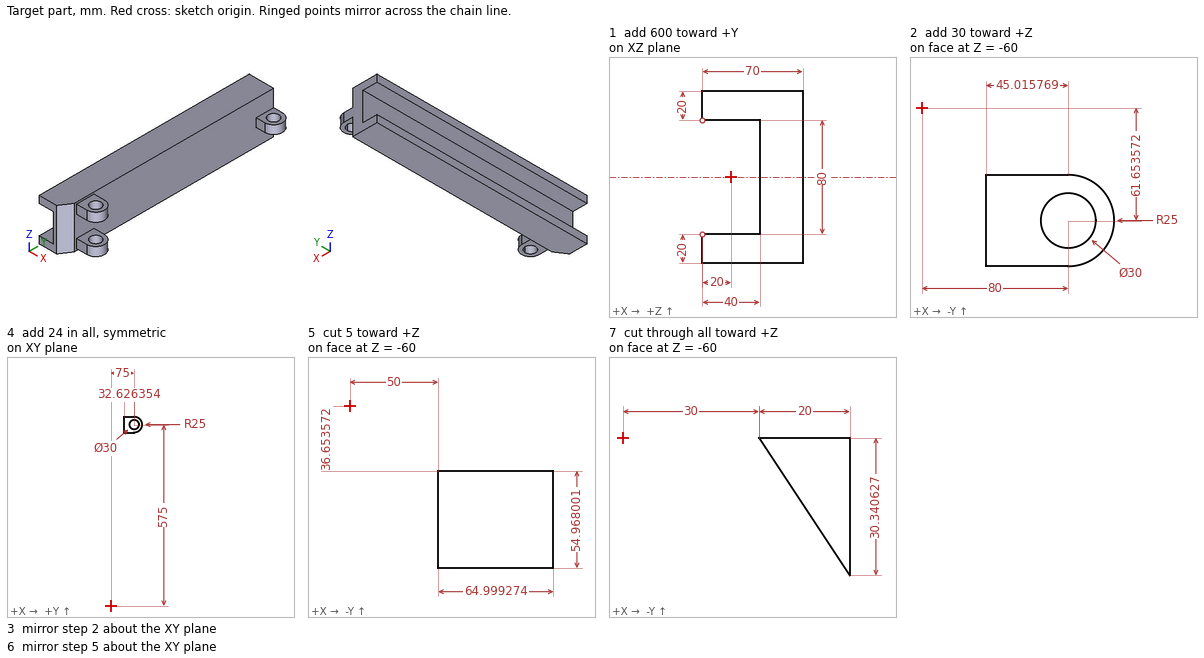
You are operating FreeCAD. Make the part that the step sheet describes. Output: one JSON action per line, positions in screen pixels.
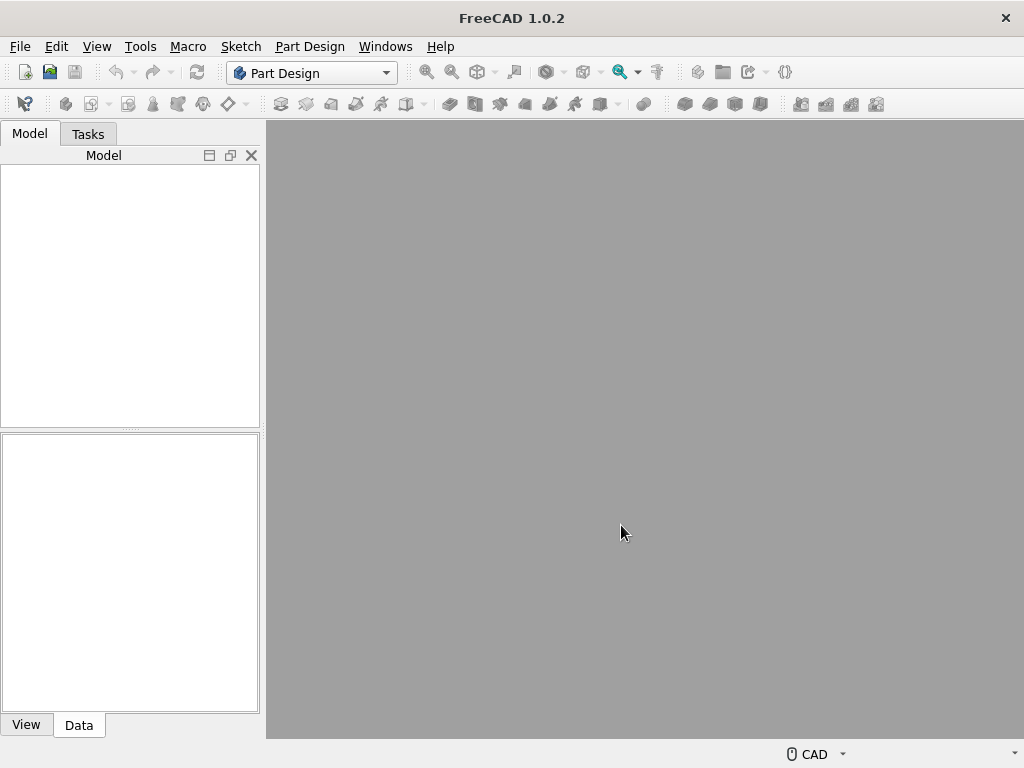
{"action": "left_click", "coordinate": [25, 72]}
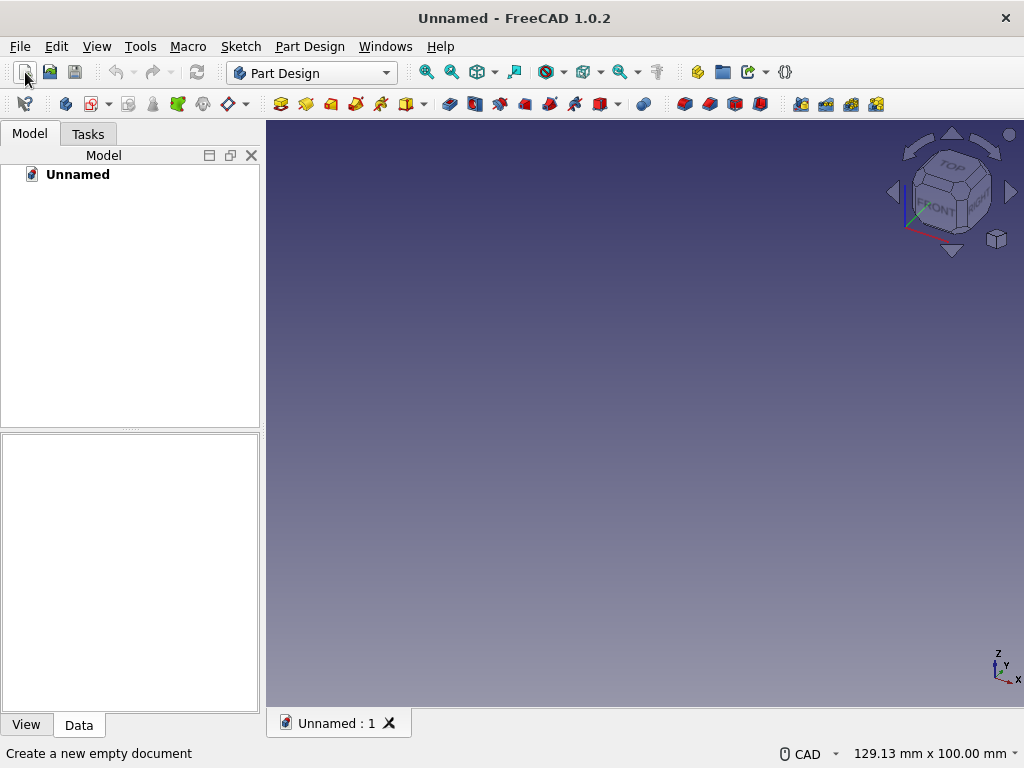
{"action": "left_click", "coordinate": [90, 104]}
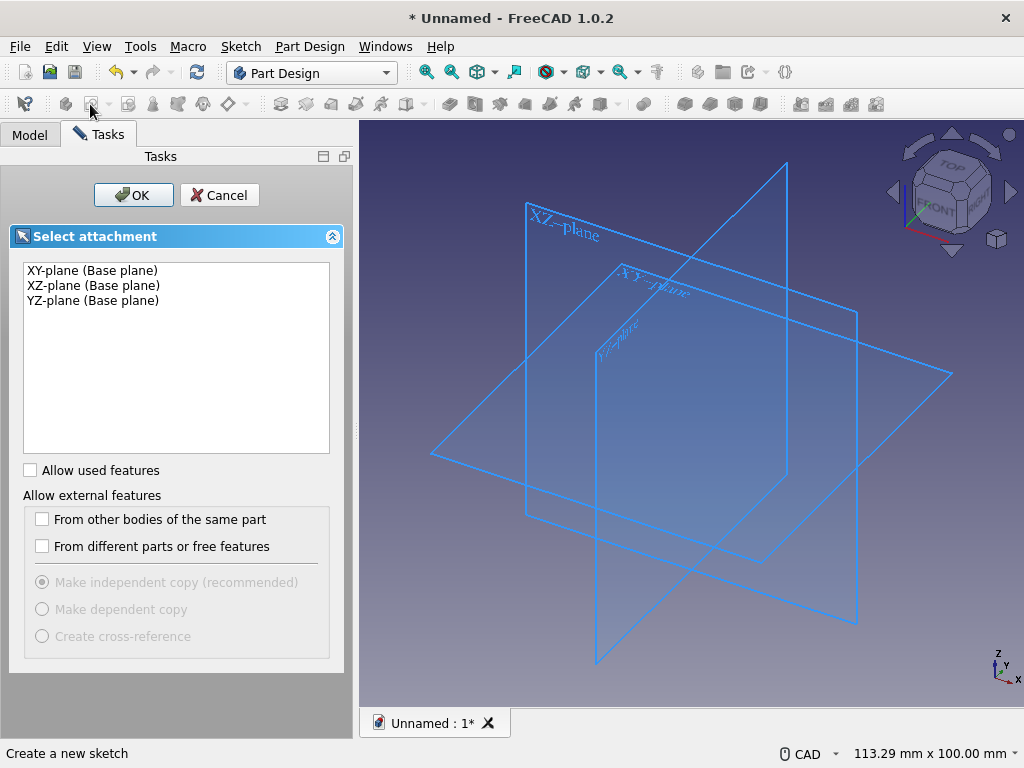
{"action": "left_click", "coordinate": [84, 286]}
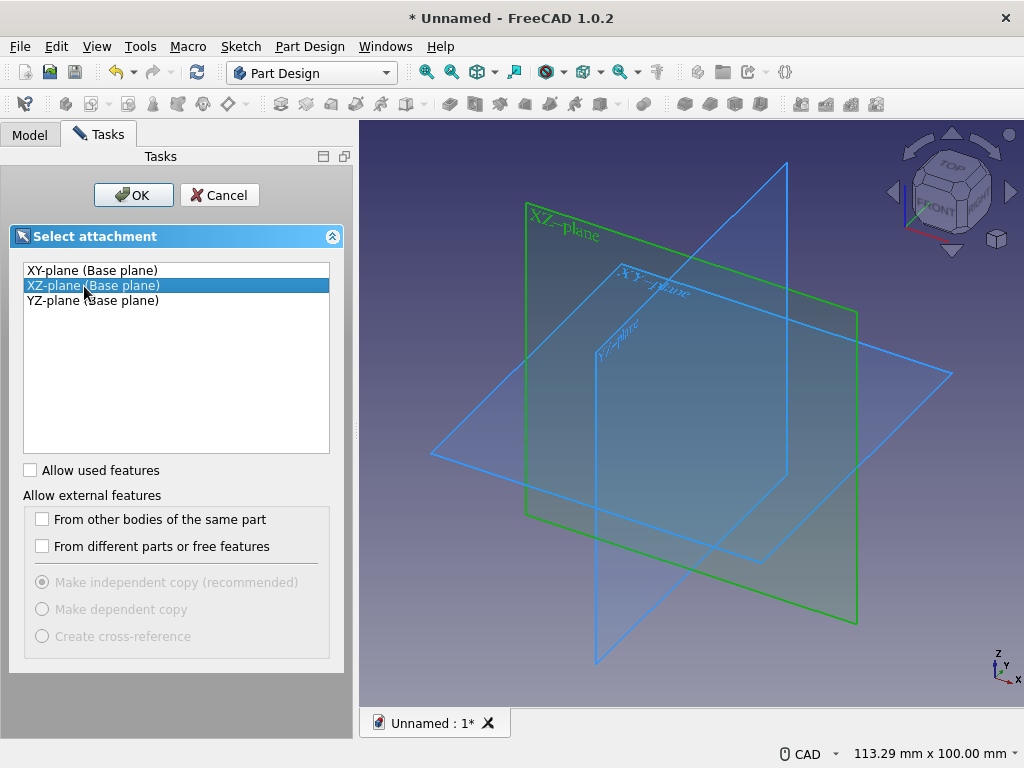
{"action": "left_click", "coordinate": [134, 195]}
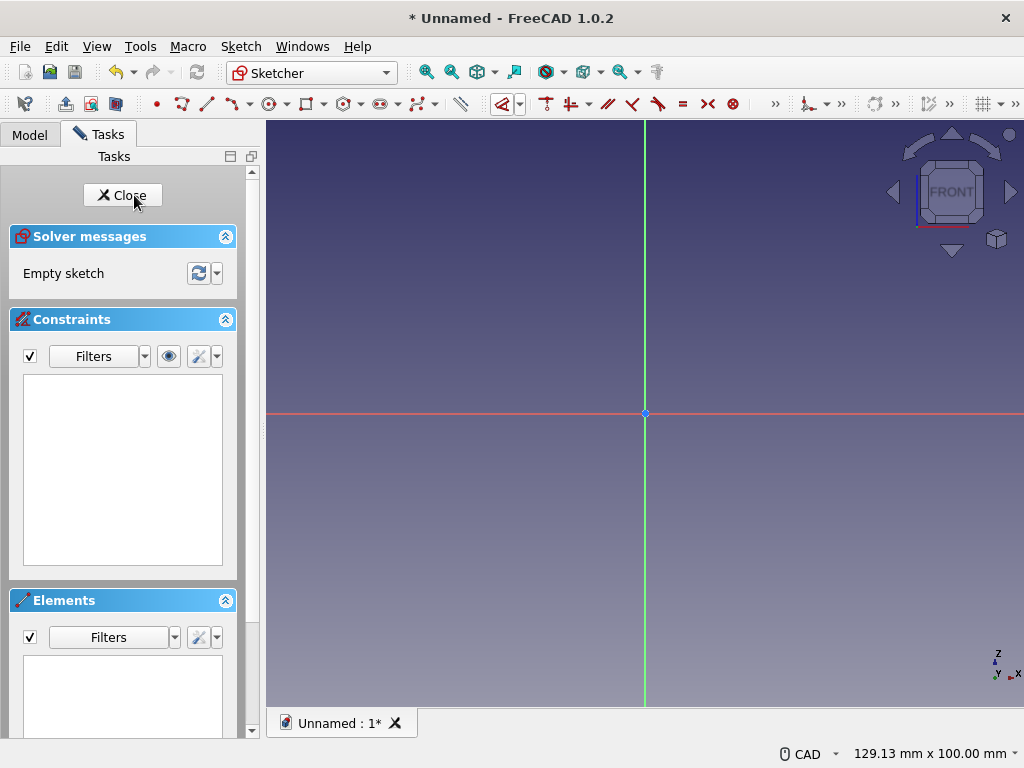
{"action": "scroll", "coordinate": [386, 414], "scroll_direction": "down", "scroll_amount": 3}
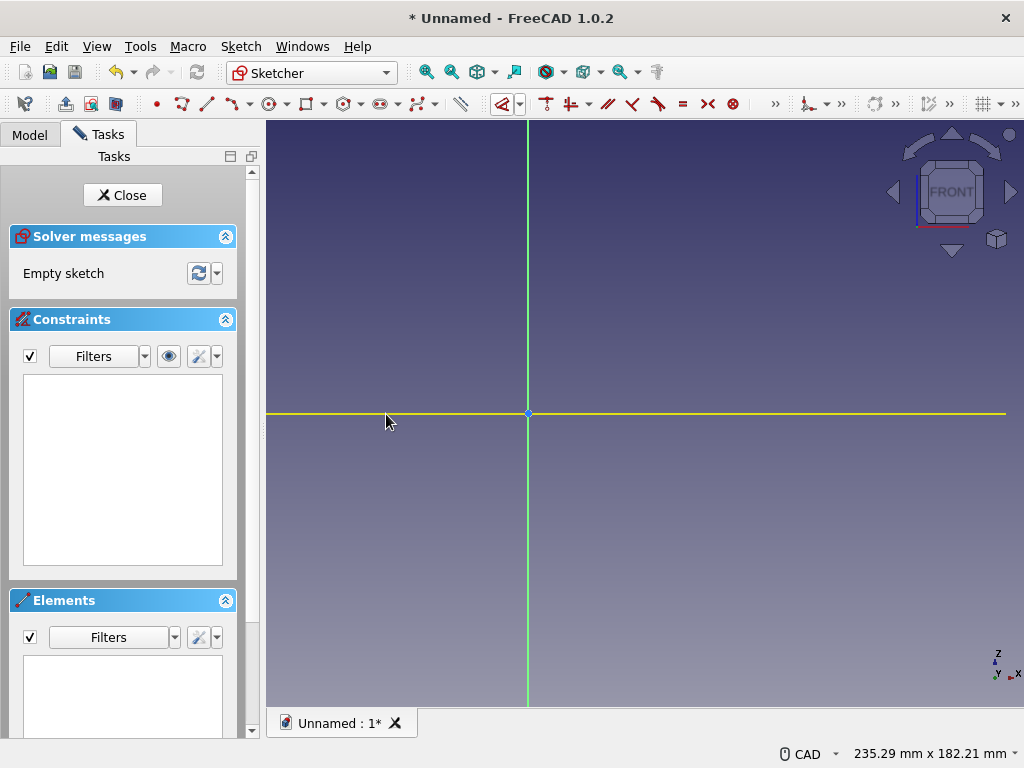
{"action": "left_click", "coordinate": [182, 104]}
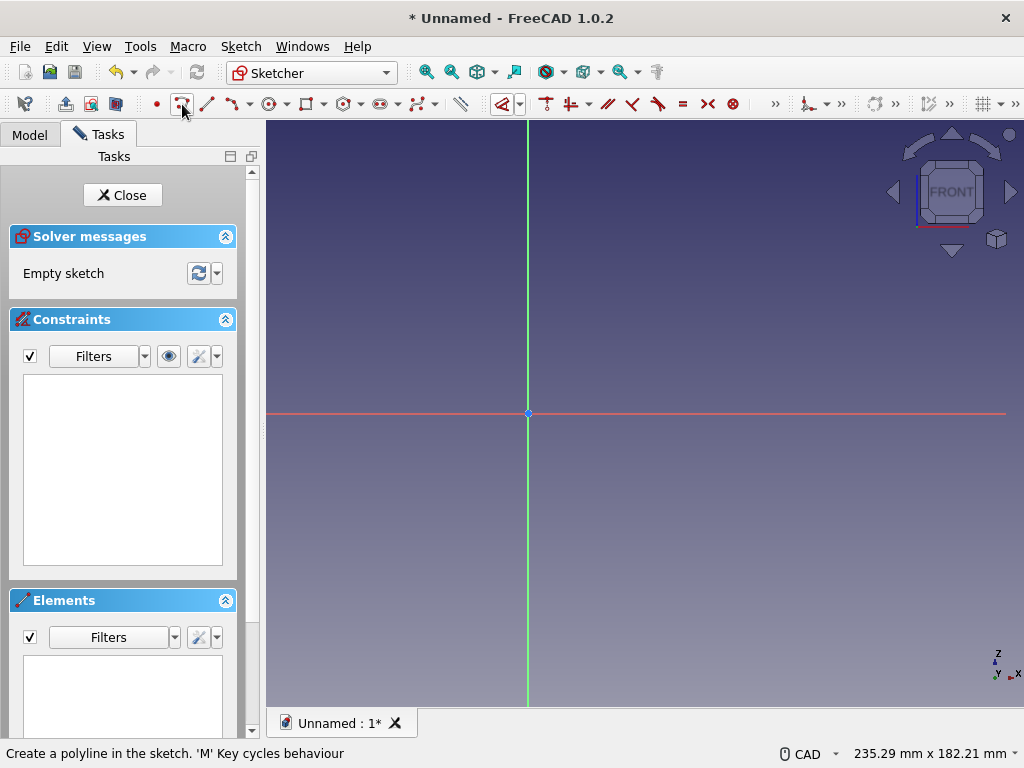
{"action": "left_click", "coordinate": [464, 543]}
{"action": "left_click", "coordinate": [593, 543]}
{"action": "left_click", "coordinate": [593, 285]}
{"action": "left_click", "coordinate": [464, 285]}
{"action": "left_click", "coordinate": [464, 221]}
{"action": "left_click", "coordinate": [689, 221]}
{"action": "left_click", "coordinate": [689, 607]}
{"action": "left_click", "coordinate": [464, 607]}
{"action": "left_click", "coordinate": [464, 544]}
{"action": "key", "text": "Escape"}
{"action": "key", "text": "Escape"}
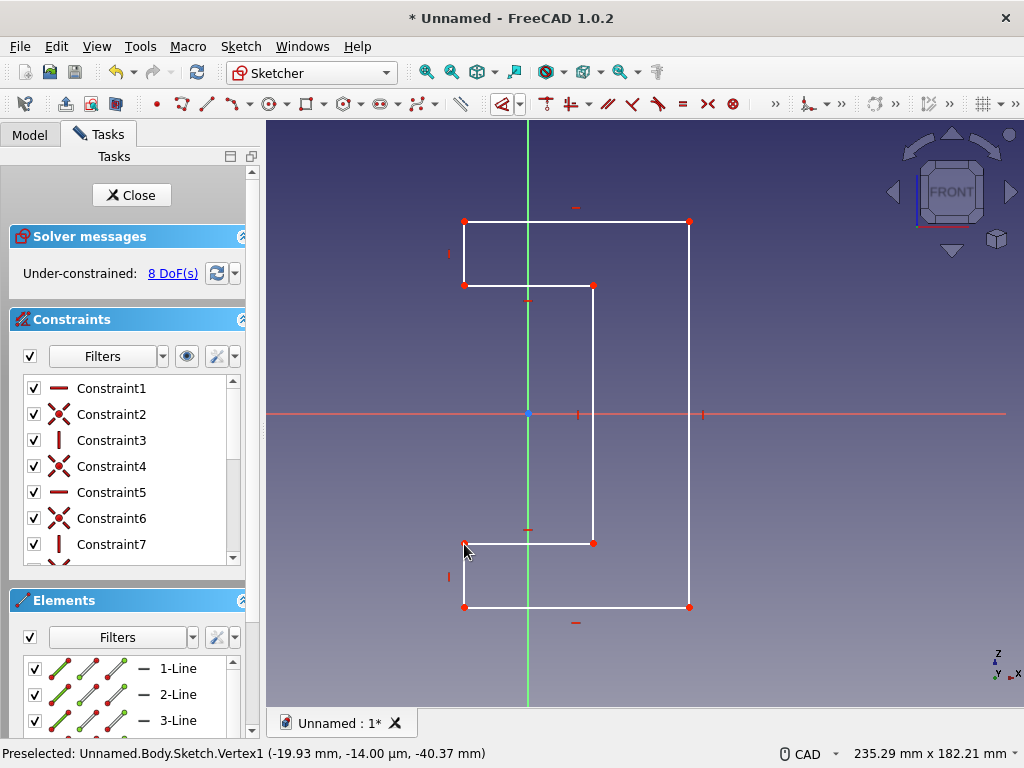
{"action": "left_click", "coordinate": [464, 544]}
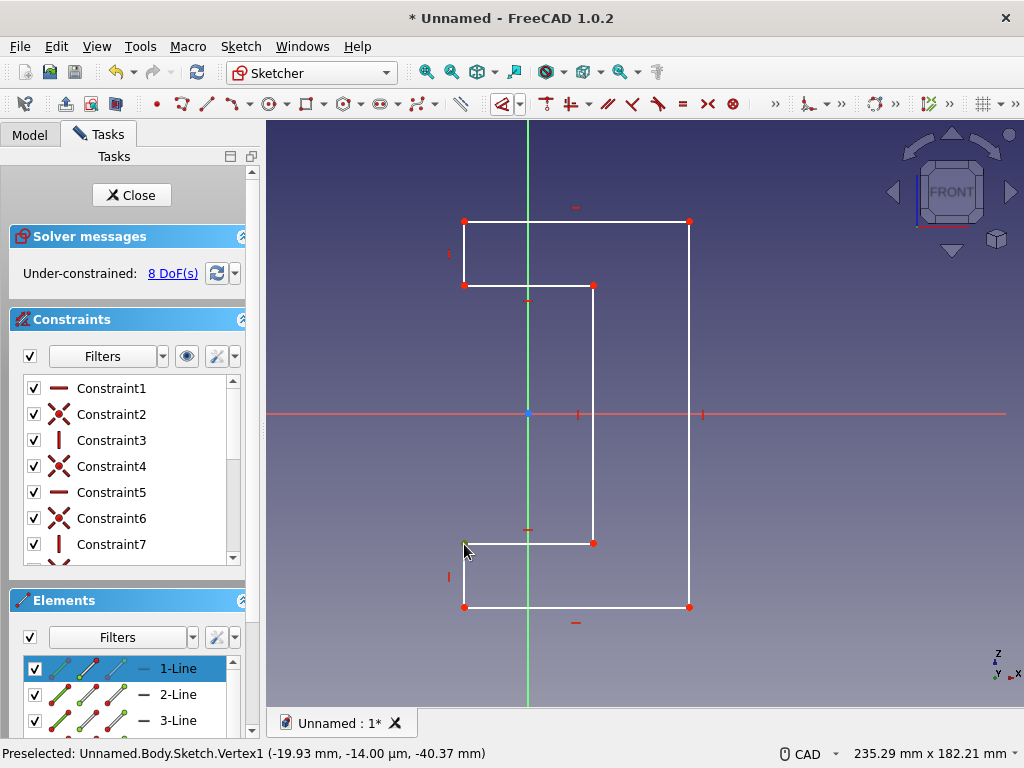
{"action": "left_click", "coordinate": [464, 286]}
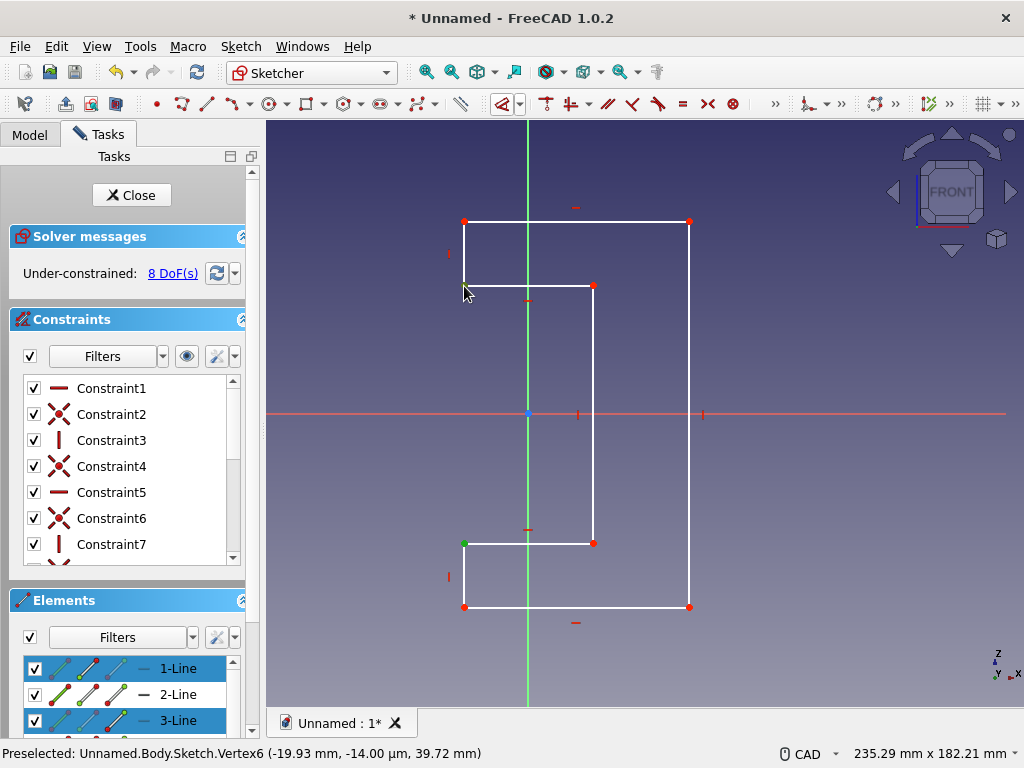
{"action": "left_click", "coordinate": [334, 414]}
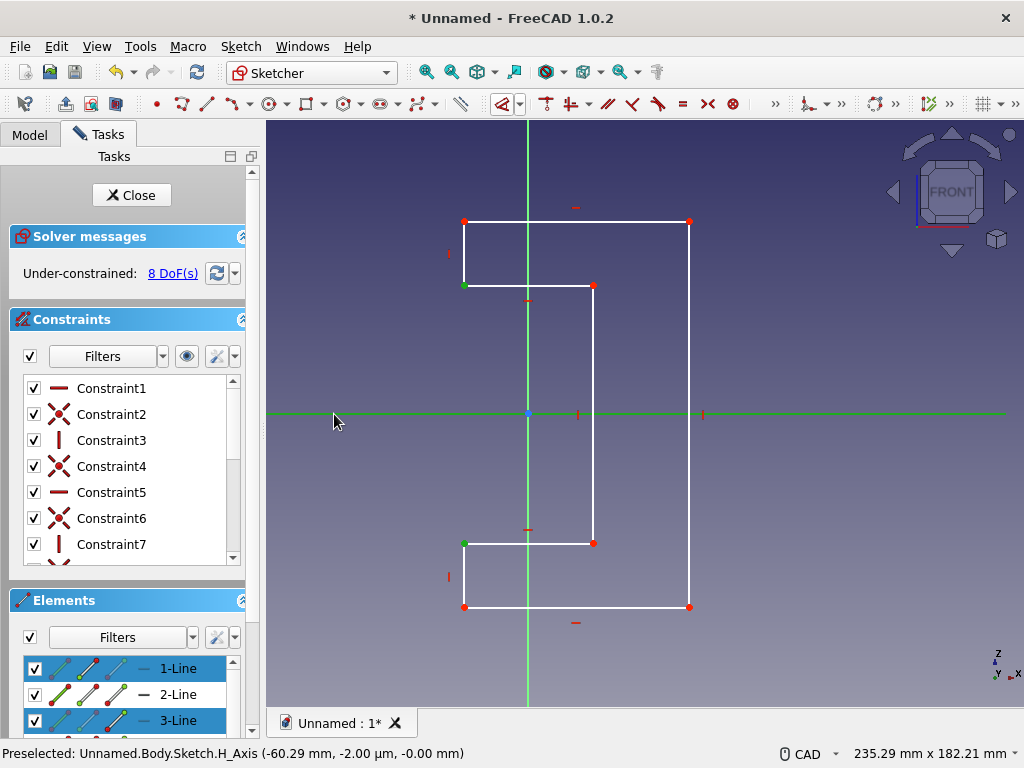
{"action": "left_click", "coordinate": [708, 104]}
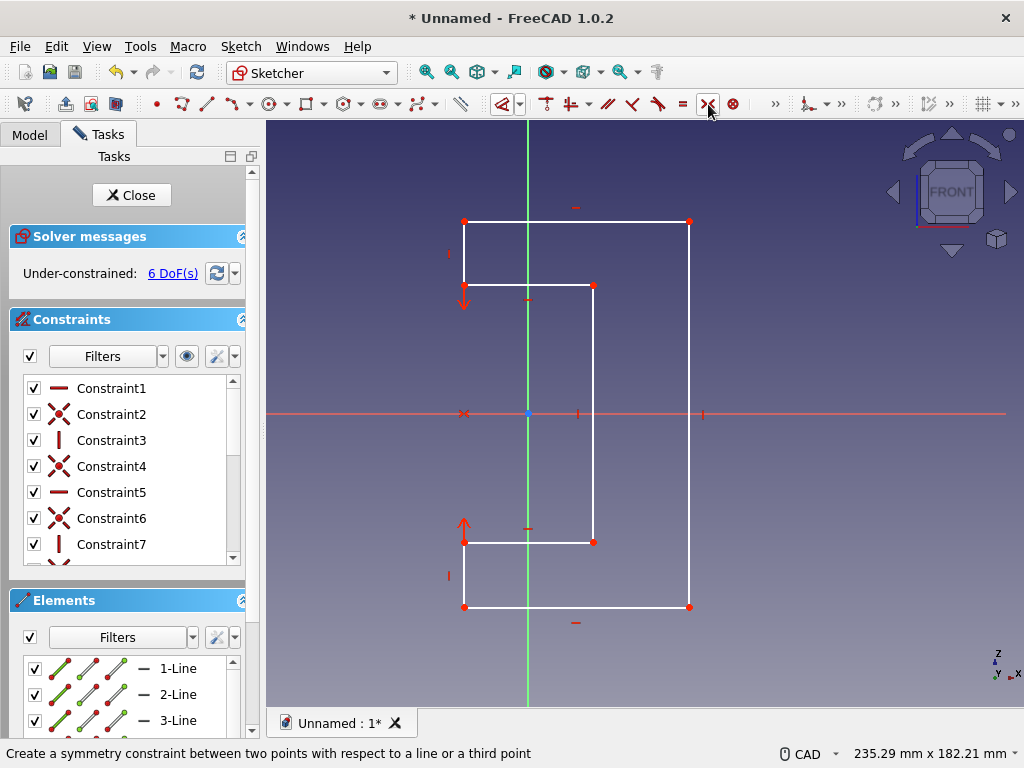
{"action": "left_click", "coordinate": [502, 104]}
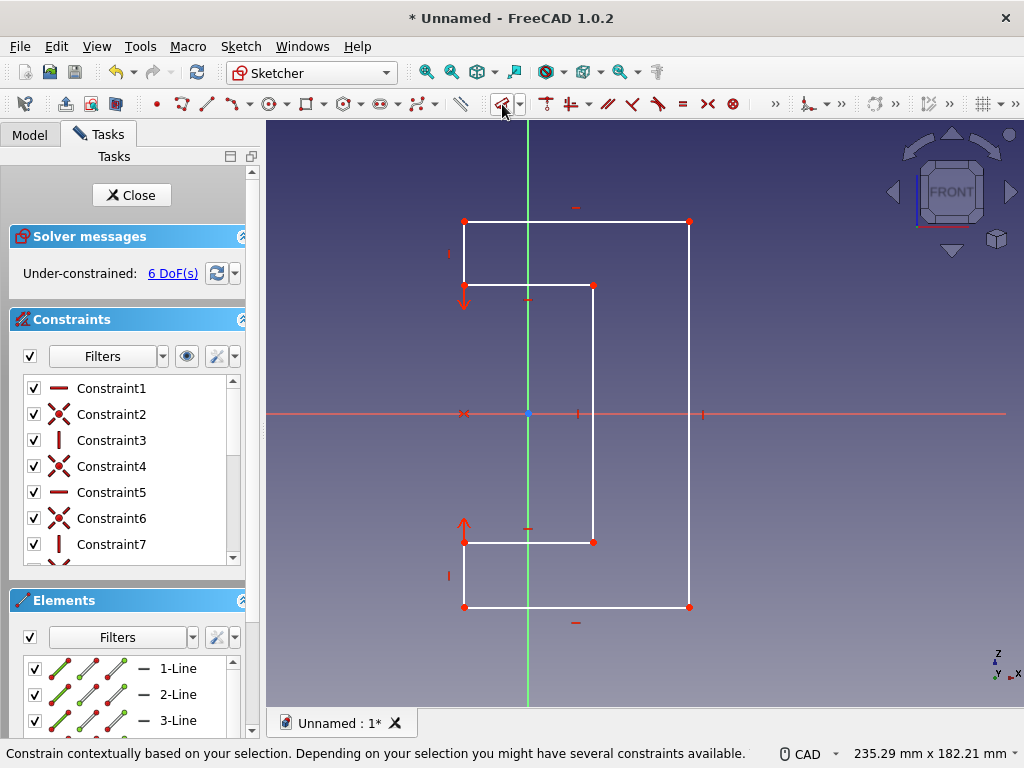
{"action": "left_click", "coordinate": [503, 543]}
{"action": "left_click", "coordinate": [499, 577]}